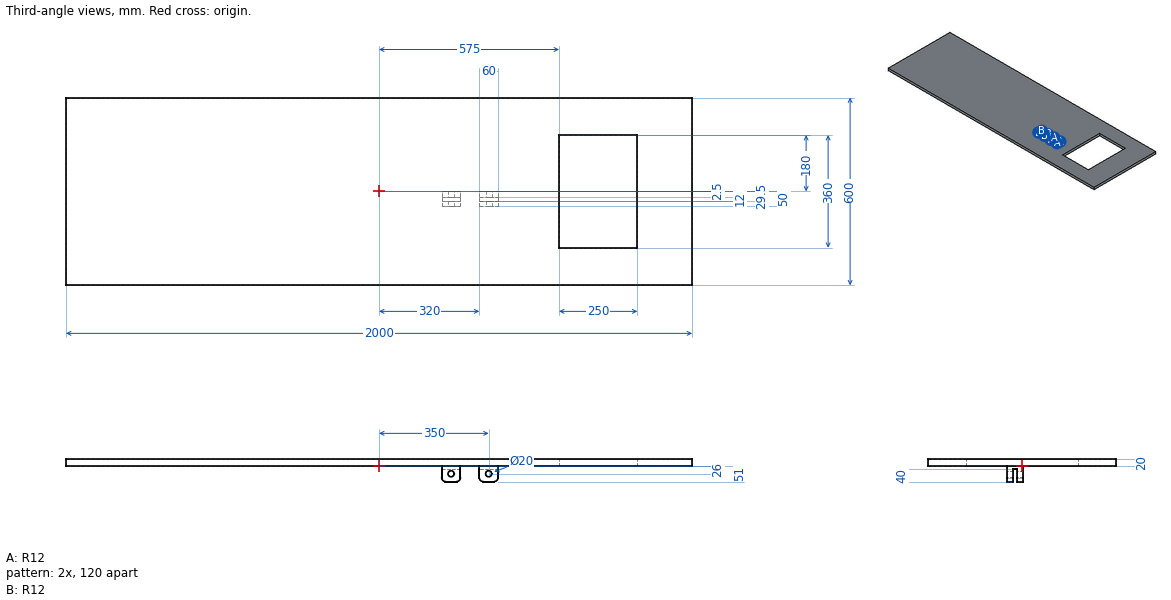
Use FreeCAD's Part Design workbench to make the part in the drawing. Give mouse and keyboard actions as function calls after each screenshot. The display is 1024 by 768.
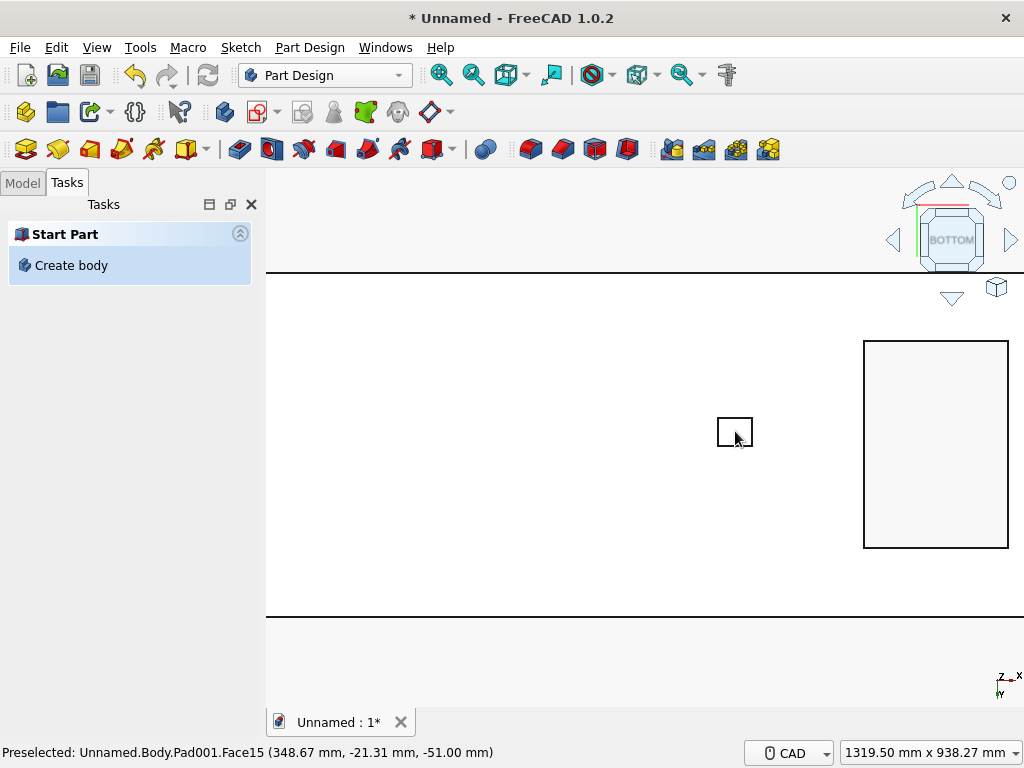
click(735, 431)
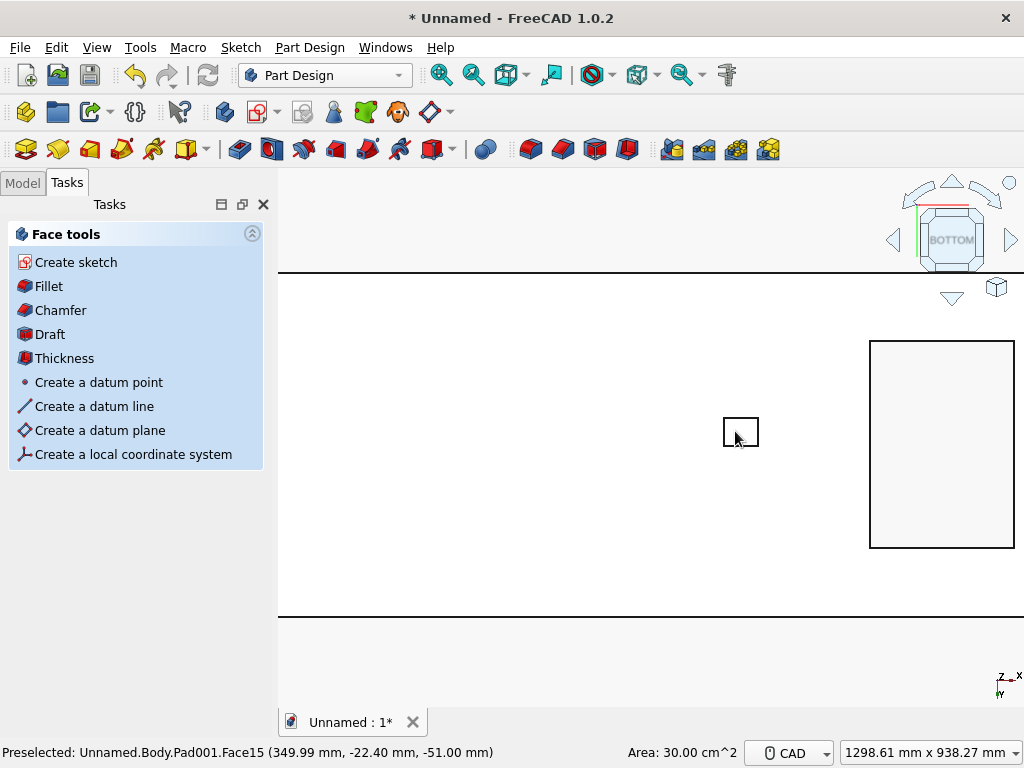
click(258, 112)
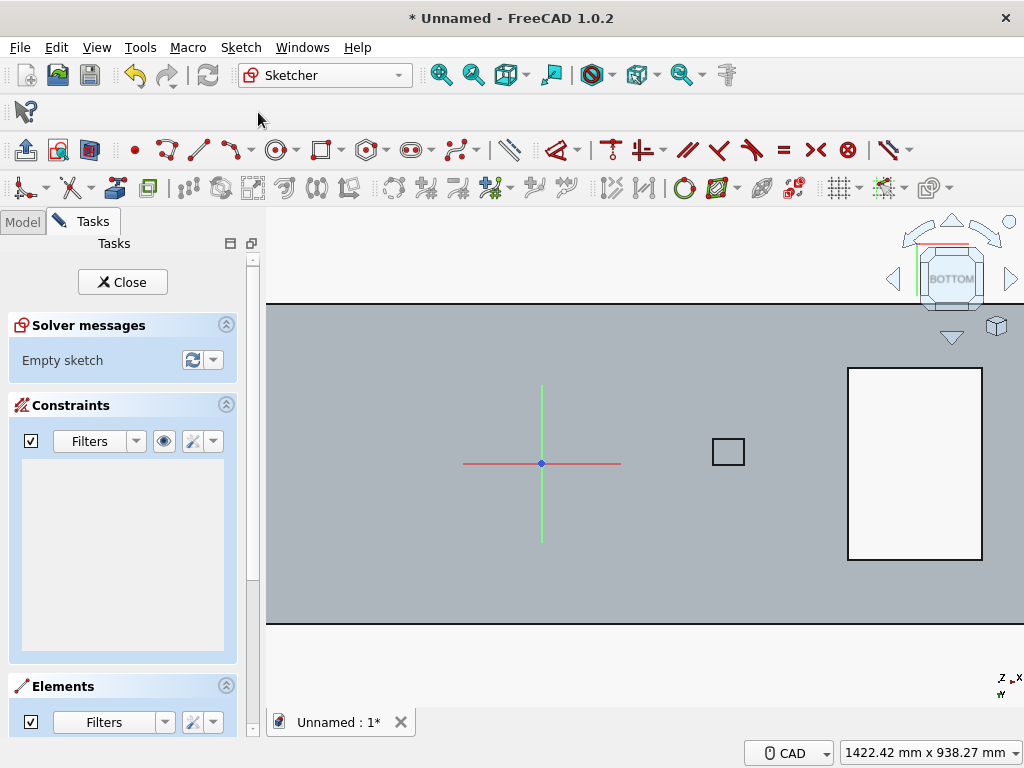
scroll(741, 451, up, 13)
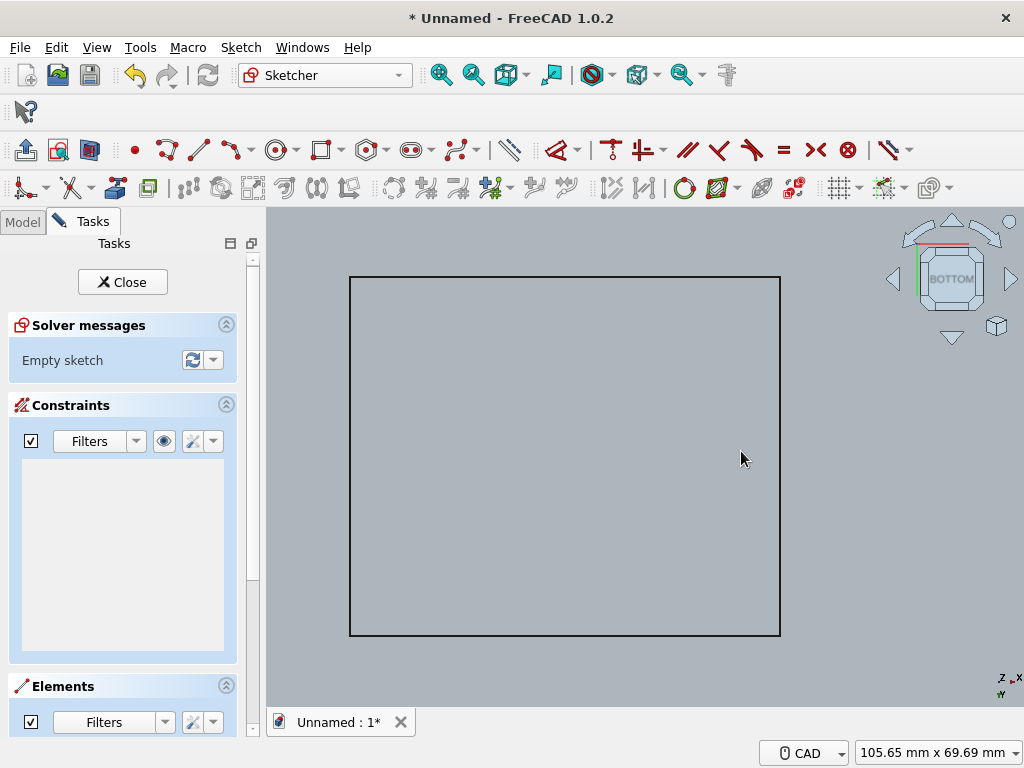
key(g)
key(r)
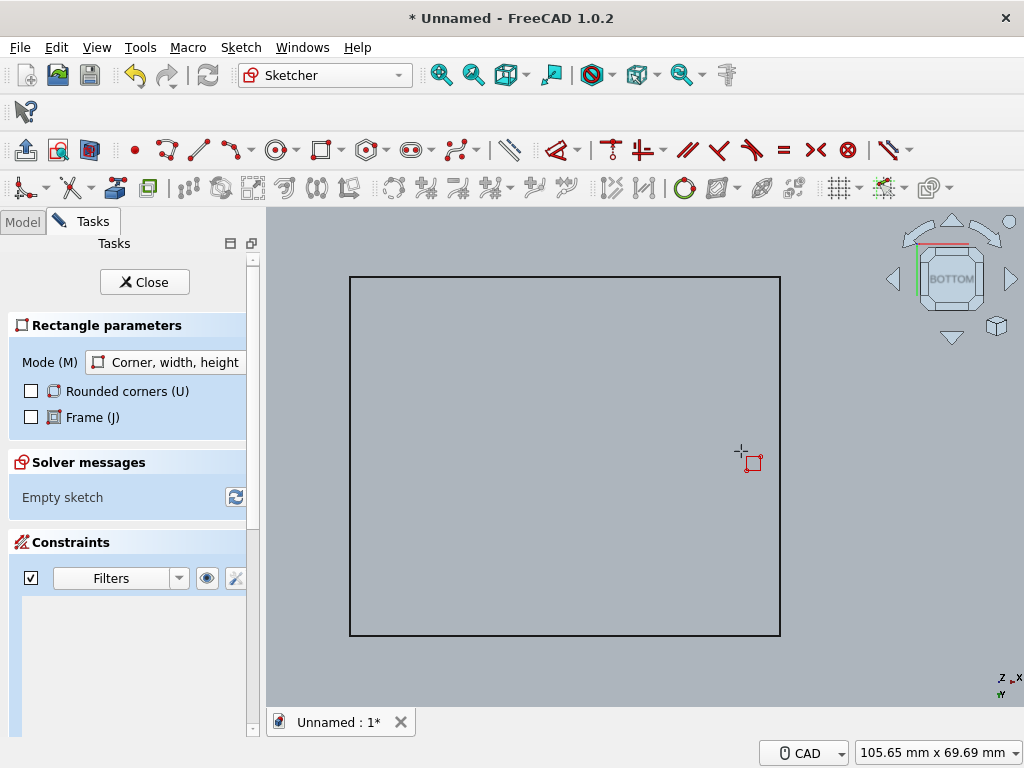
click(350, 406)
move(780, 492)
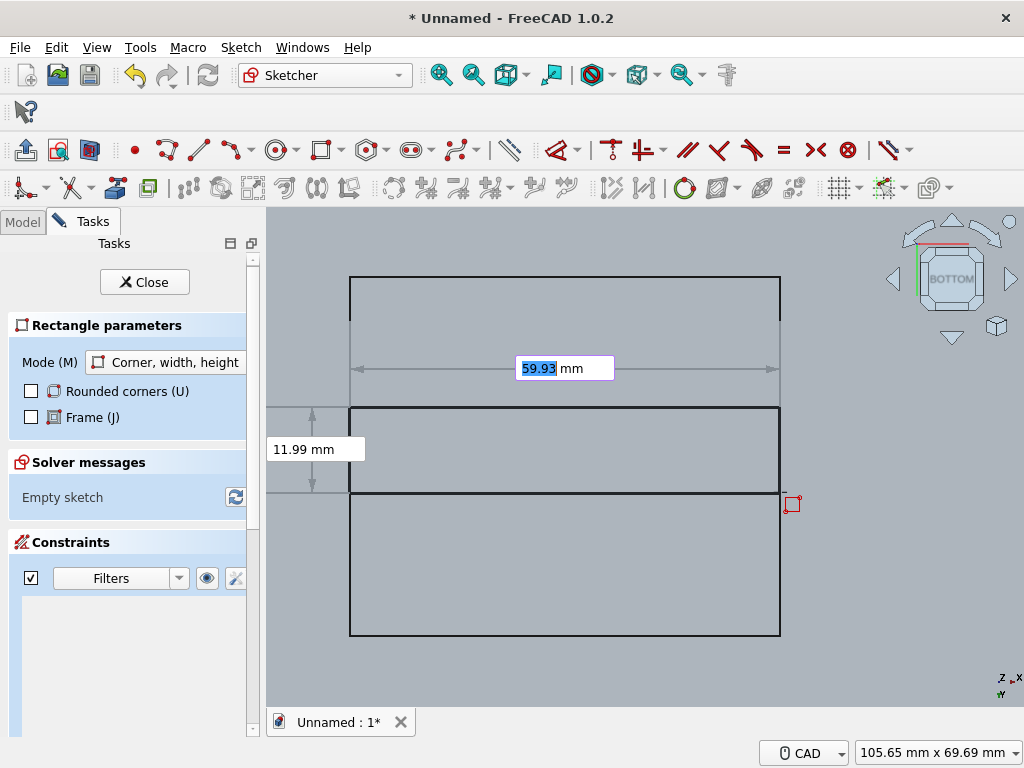
text(60)
key(Tab)
text(12)
key(Return)
key(Escape)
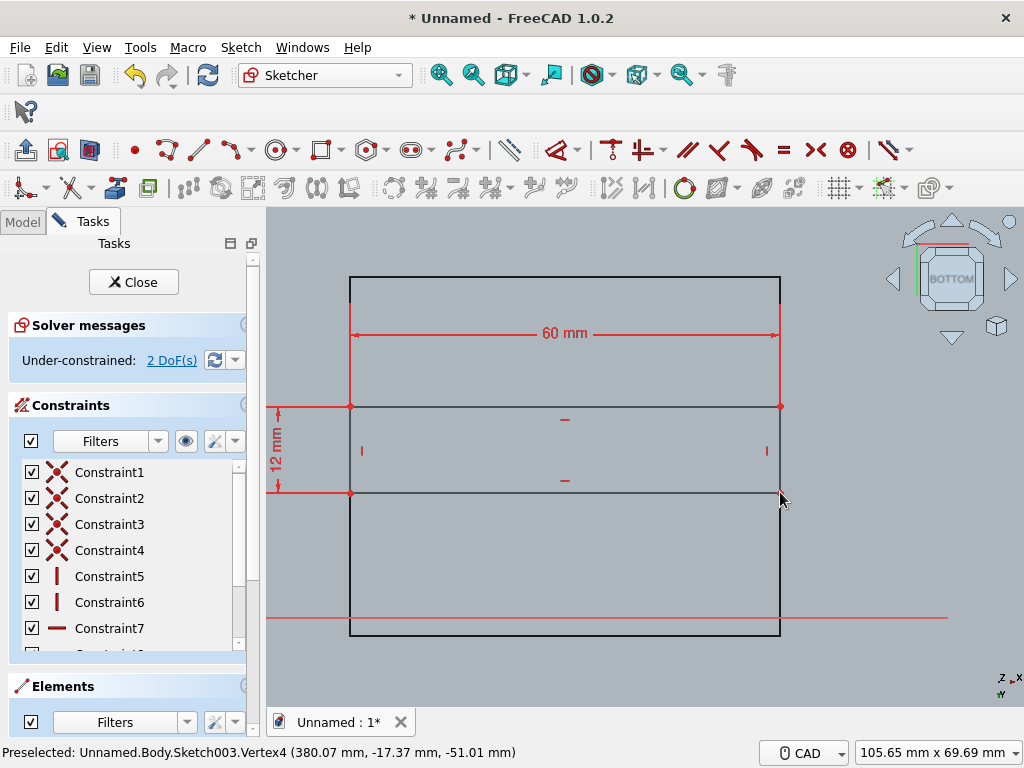
key(d)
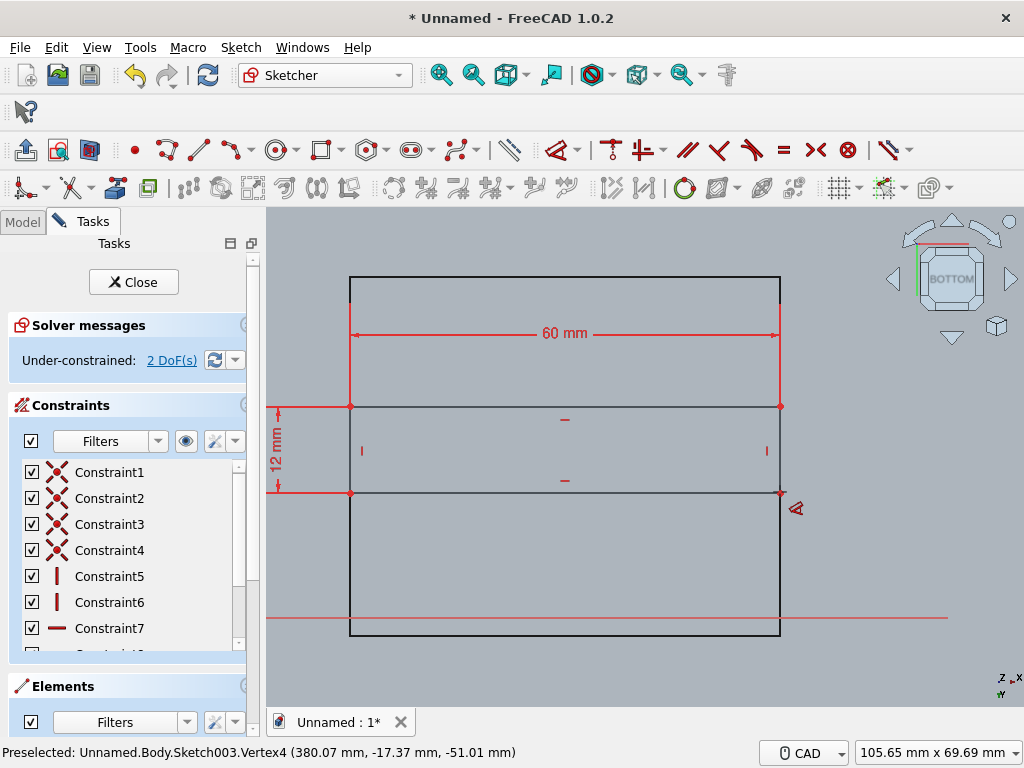
click(350, 407)
click(322, 652)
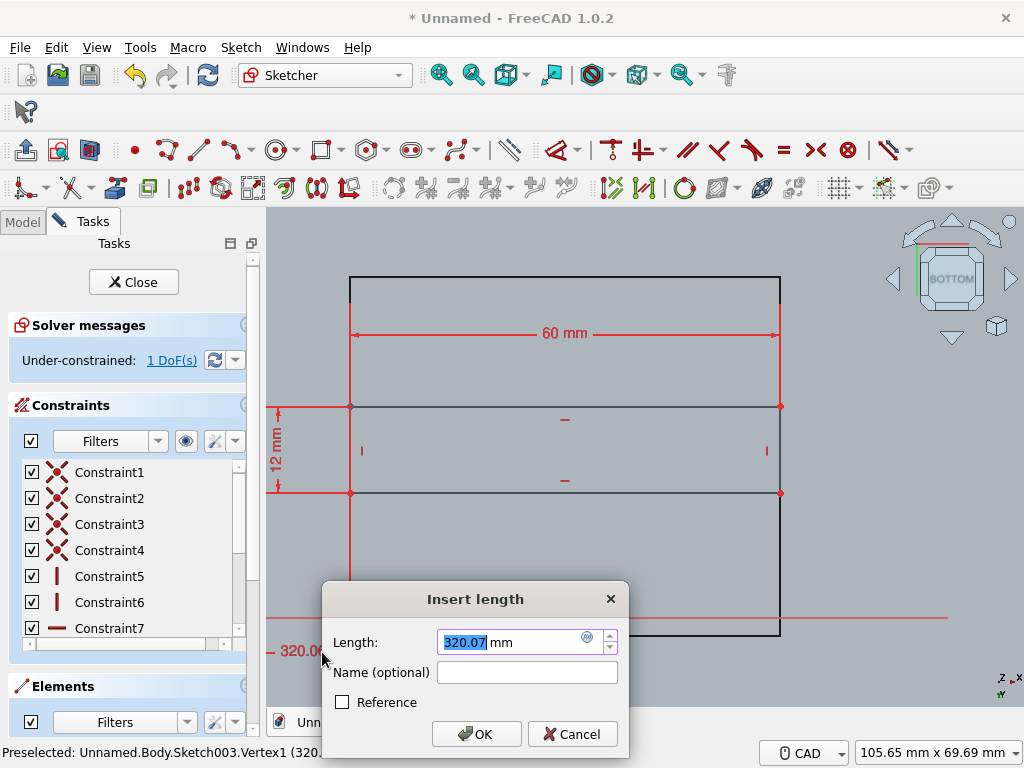
text(320)
key(Return)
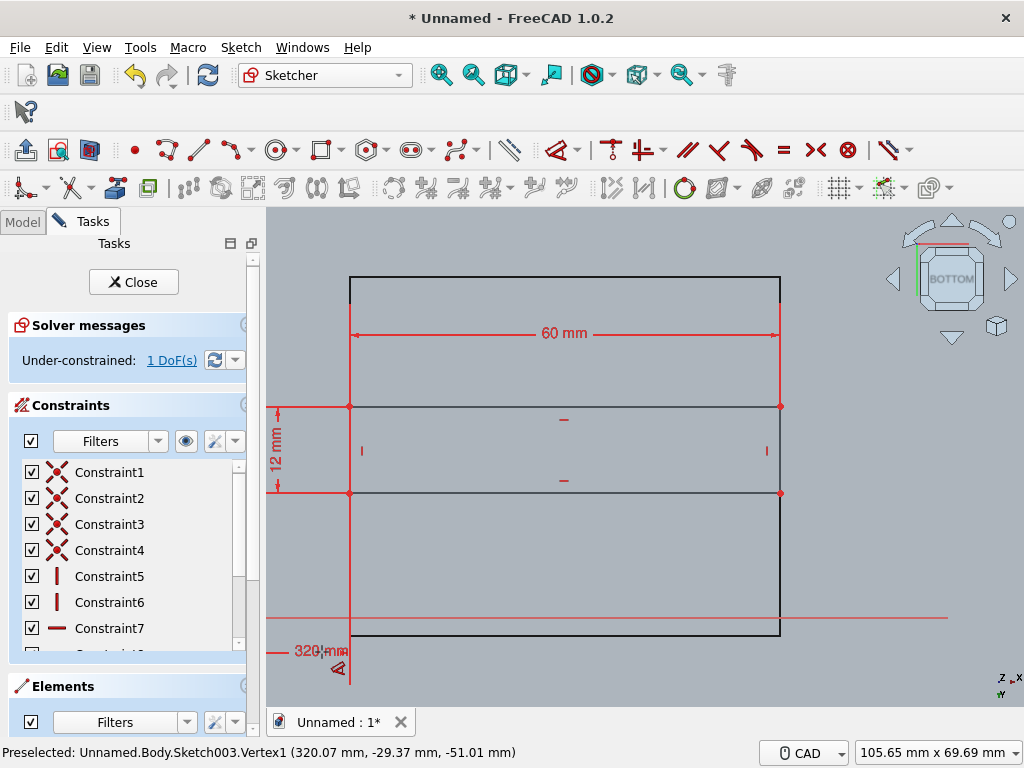
click(350, 407)
click(384, 512)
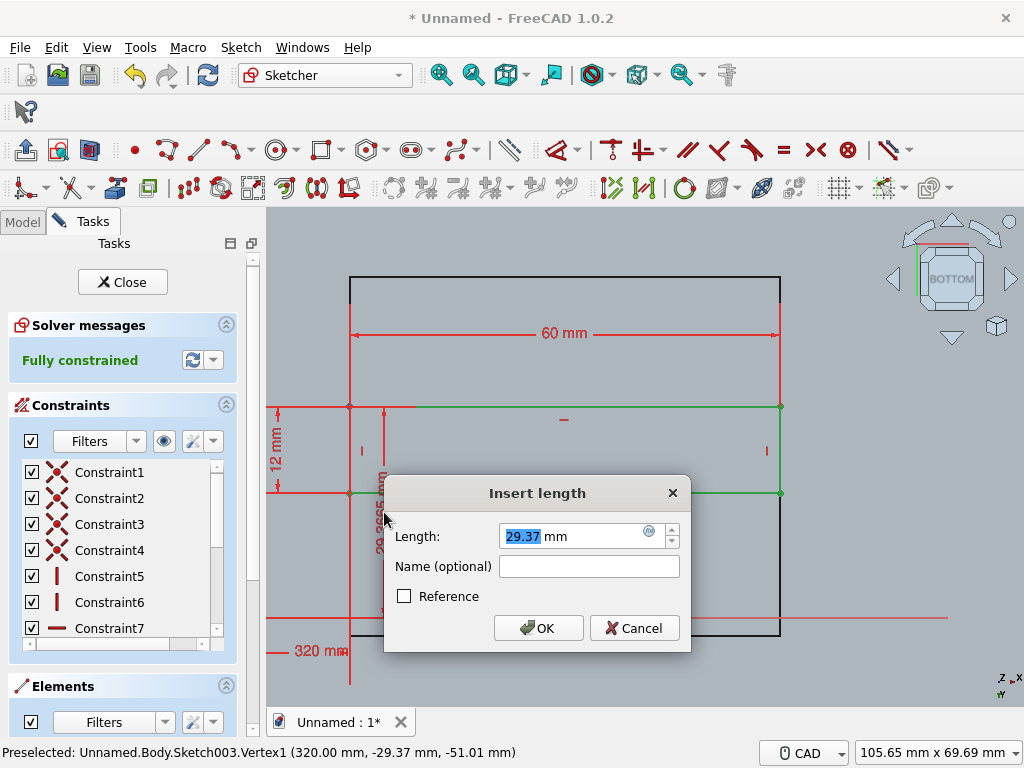
text(29.5)
key(Return)
key(Escape)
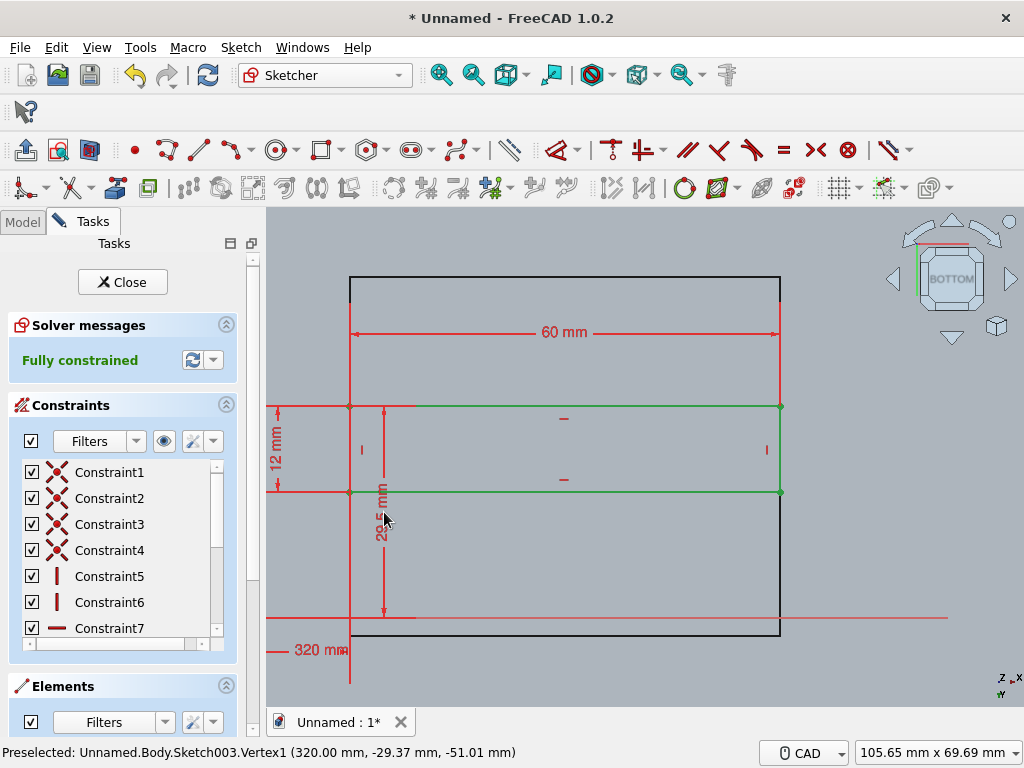
click(123, 282)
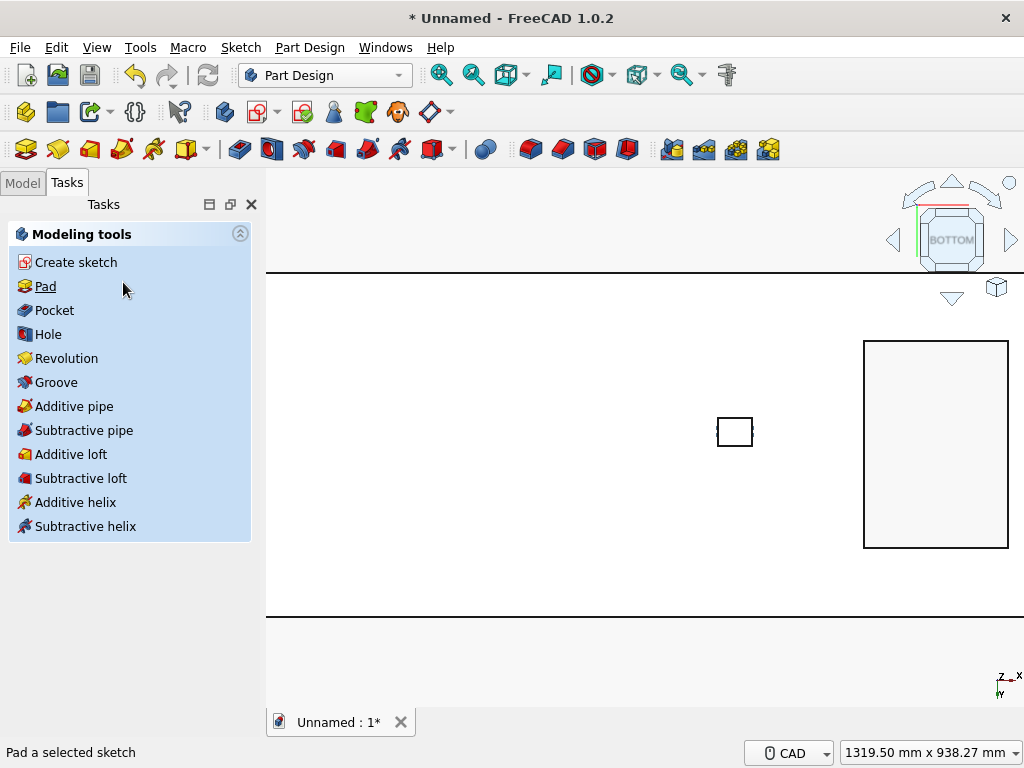
click(240, 150)